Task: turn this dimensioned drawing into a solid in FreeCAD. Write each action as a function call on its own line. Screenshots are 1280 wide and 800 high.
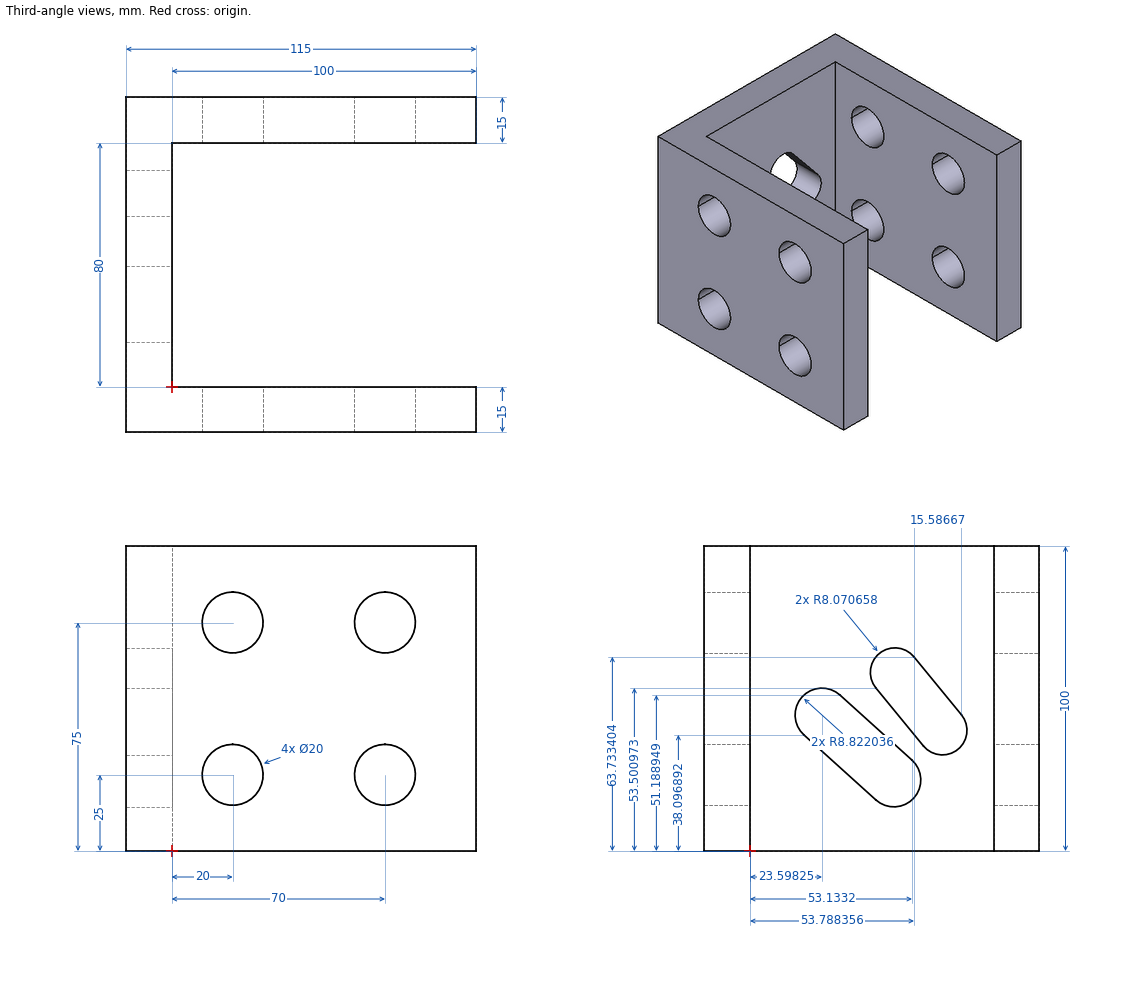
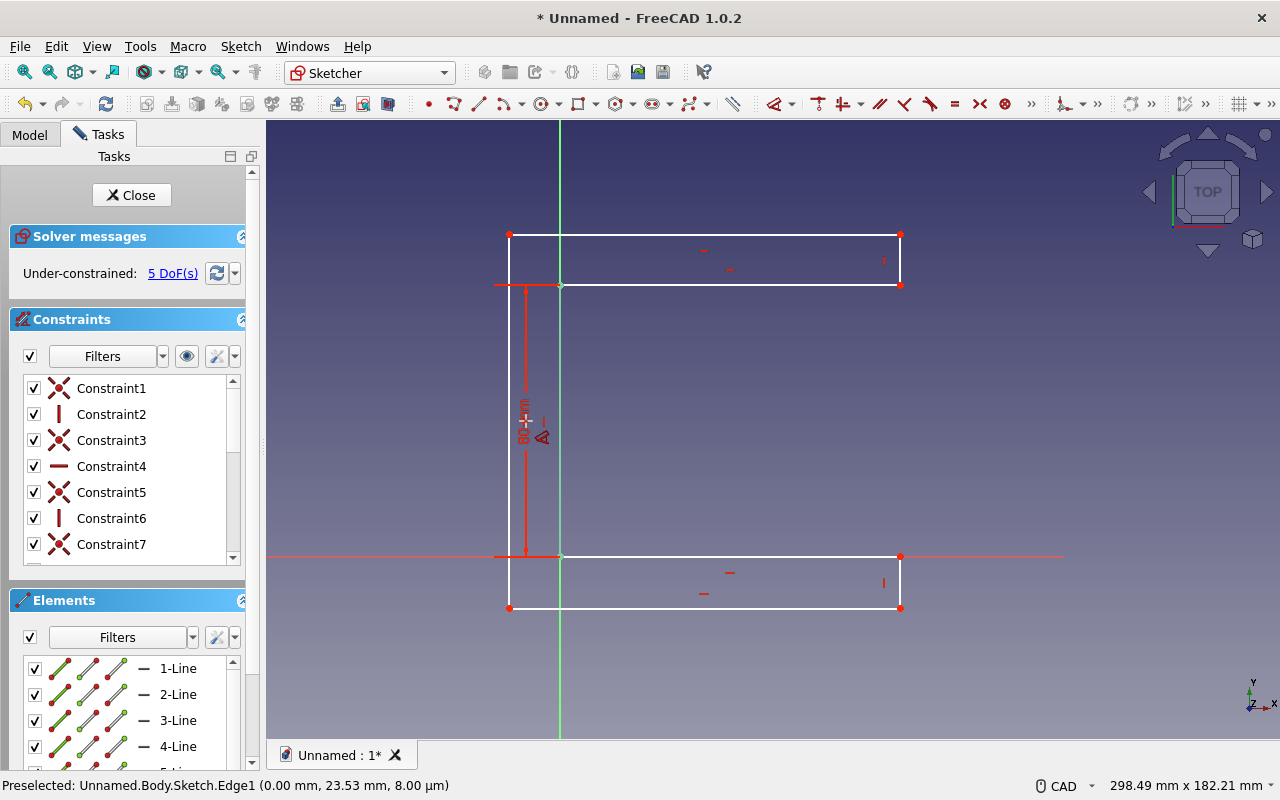
click(900, 270)
click(934, 260)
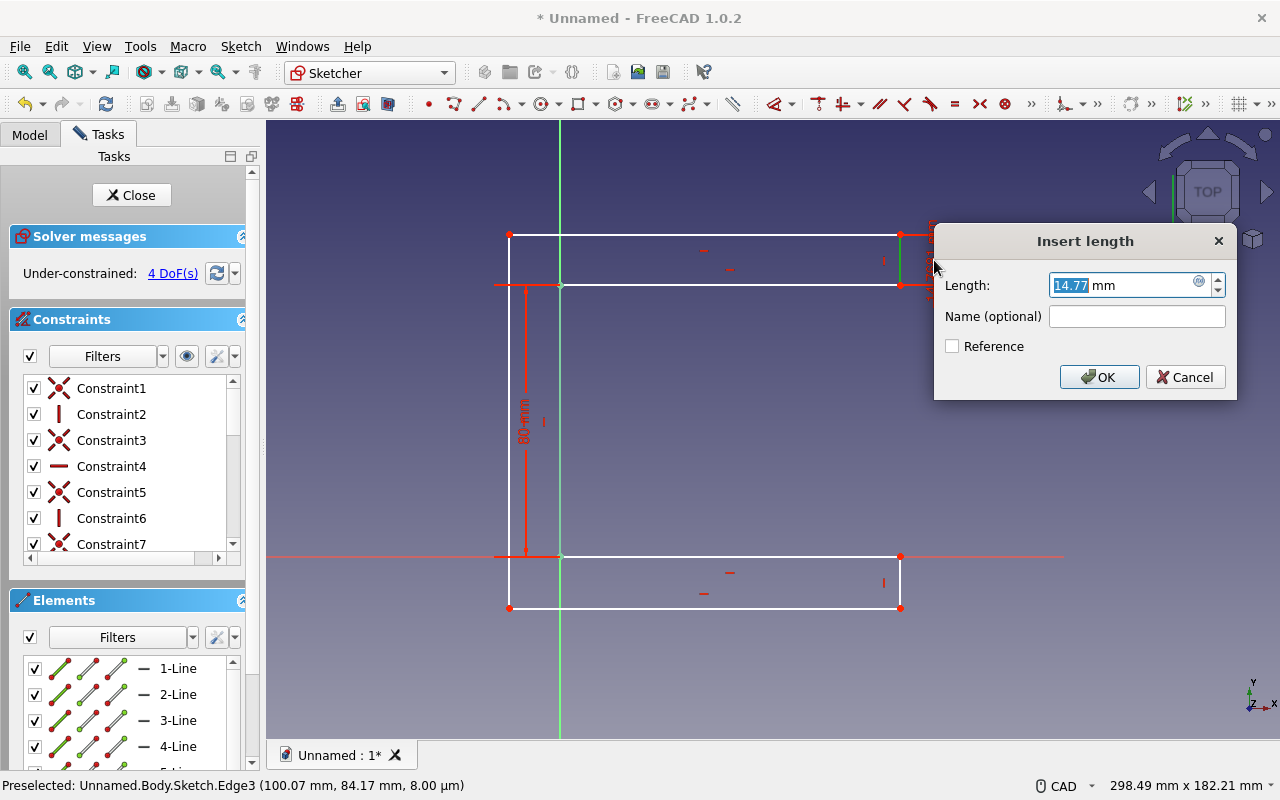
text(15)
key(Return)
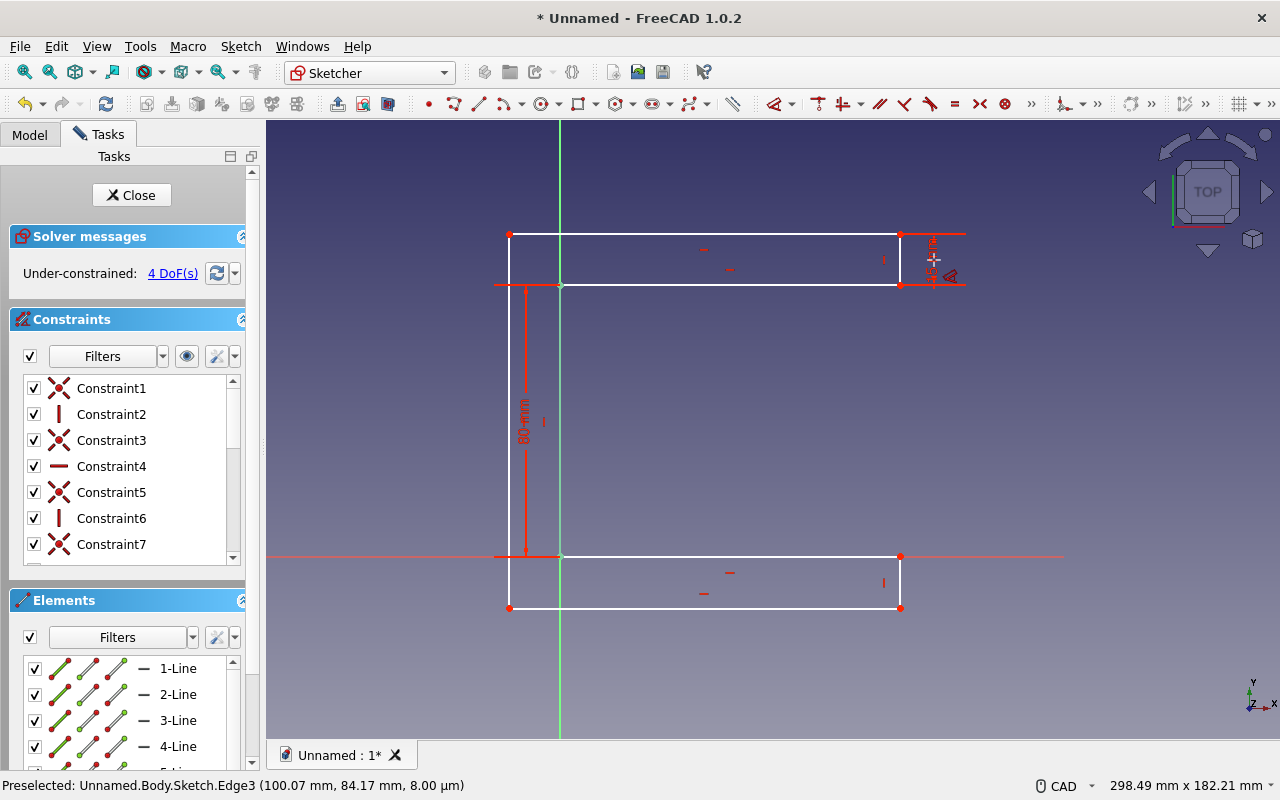
click(900, 593)
click(934, 583)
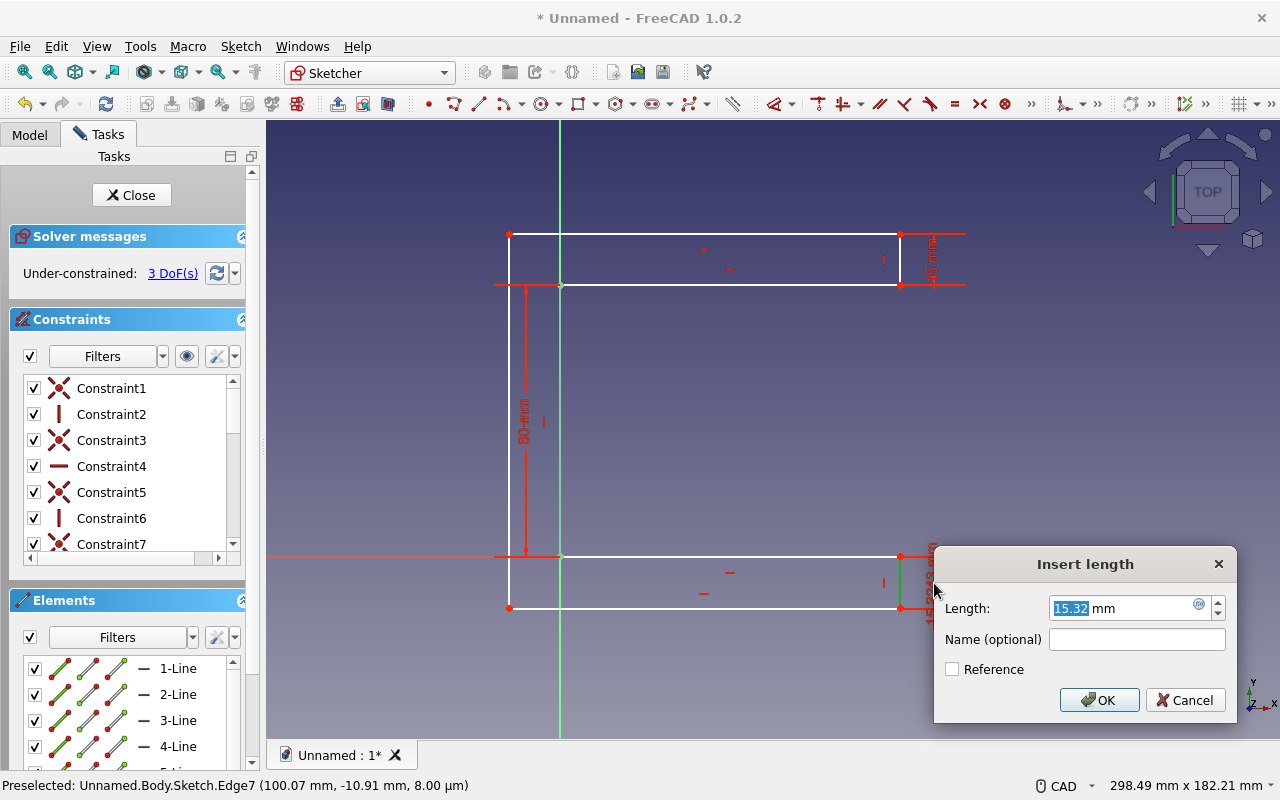
text(15)
key(Return)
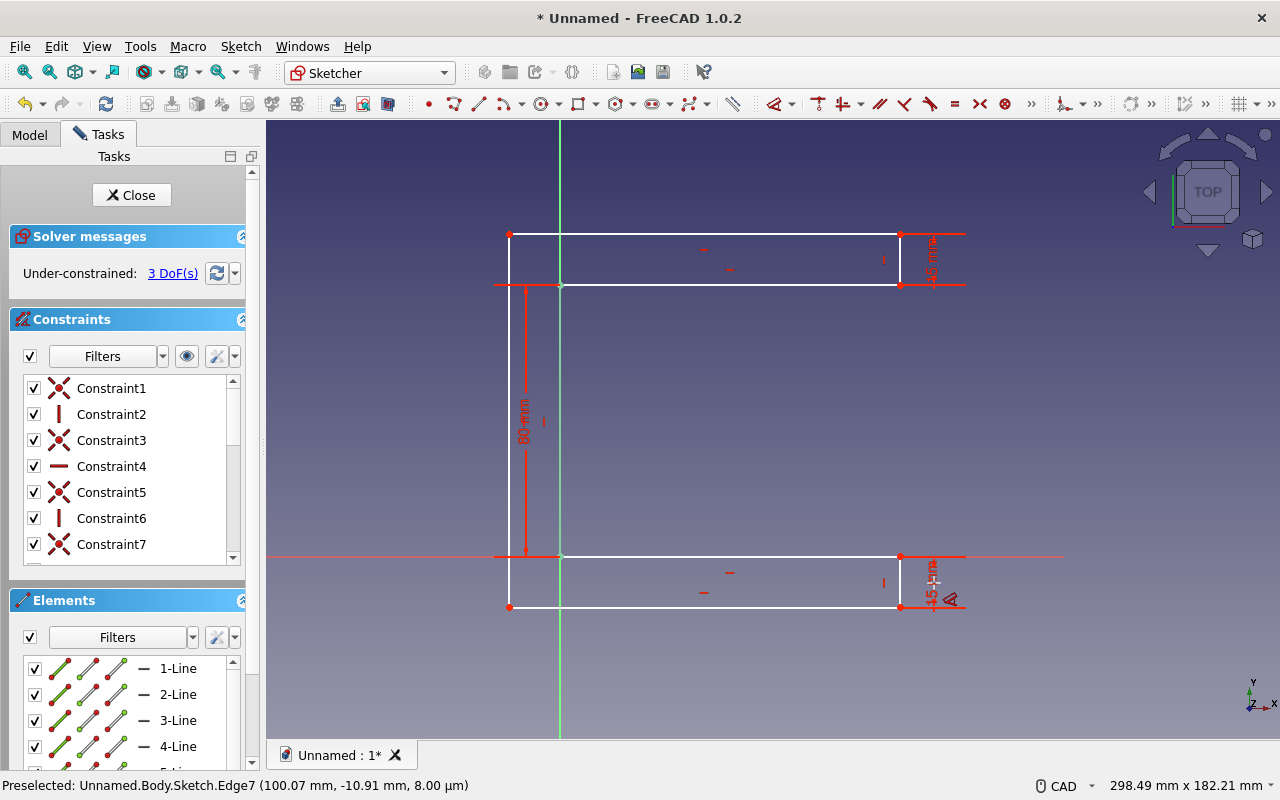
click(662, 285)
click(730, 251)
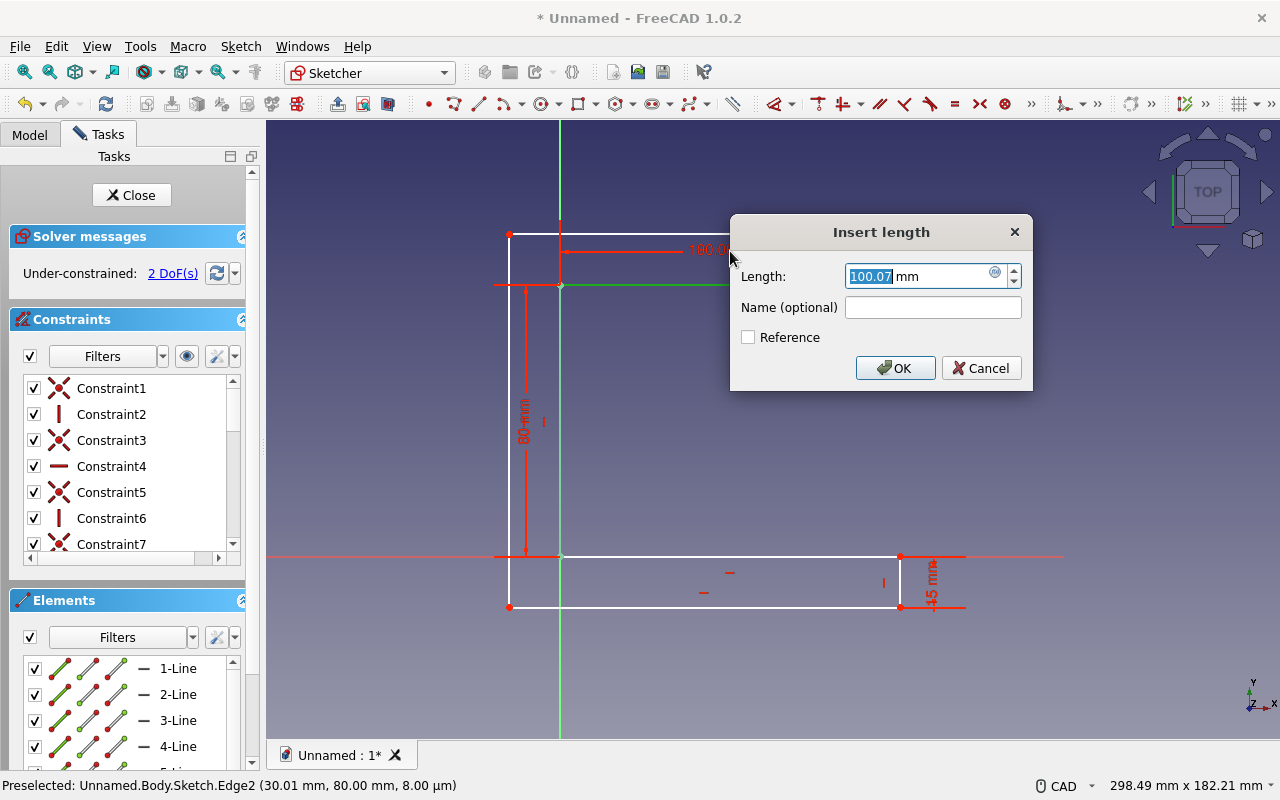
text(100)
key(Return)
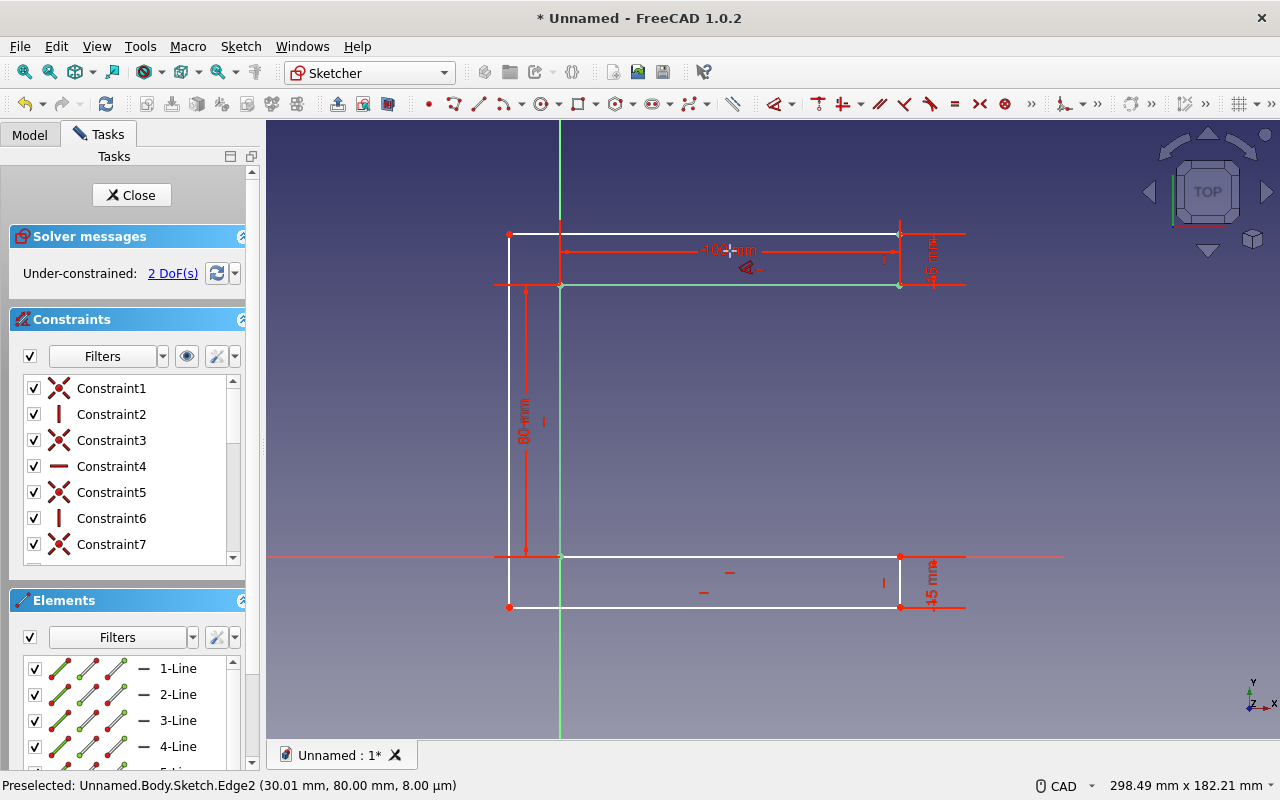
click(783, 234)
click(704, 200)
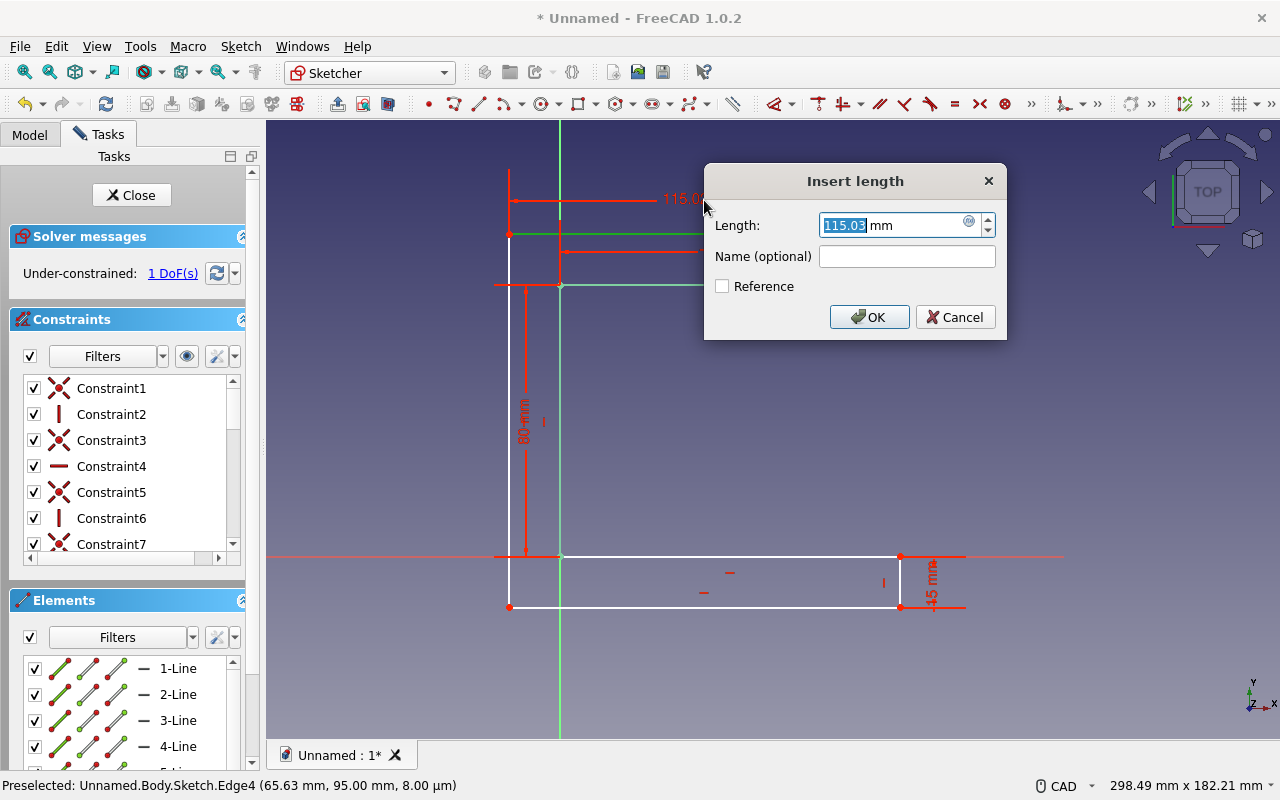
text(115)
key(Return)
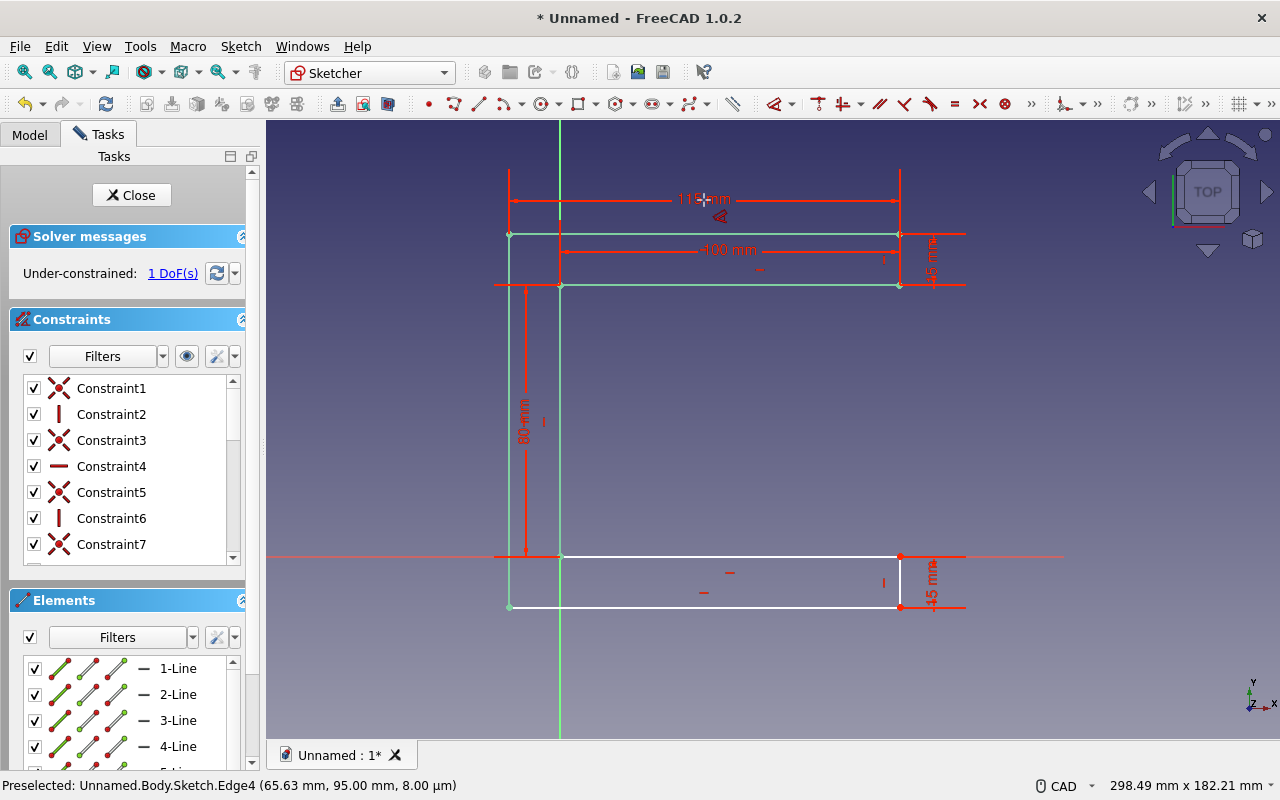
click(626, 608)
click(705, 642)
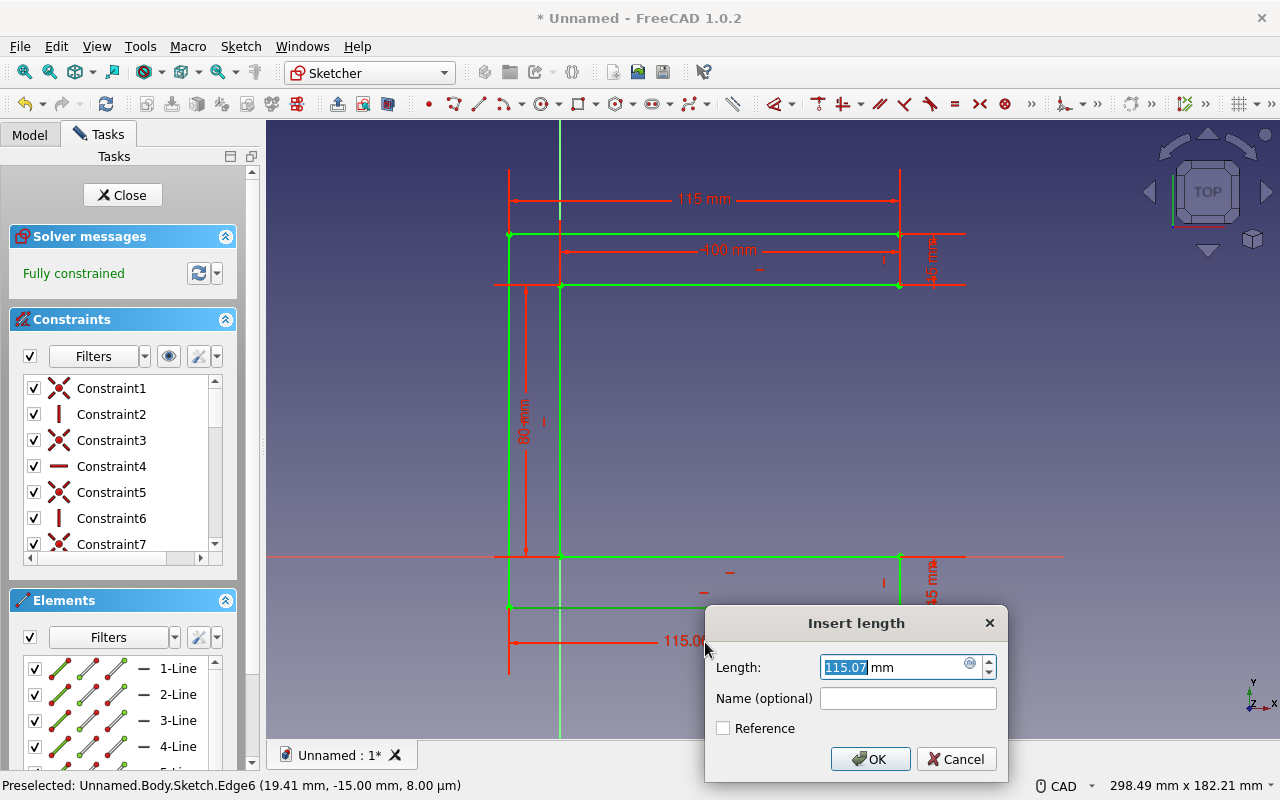
text(115)
key(Return)
key(Escape)